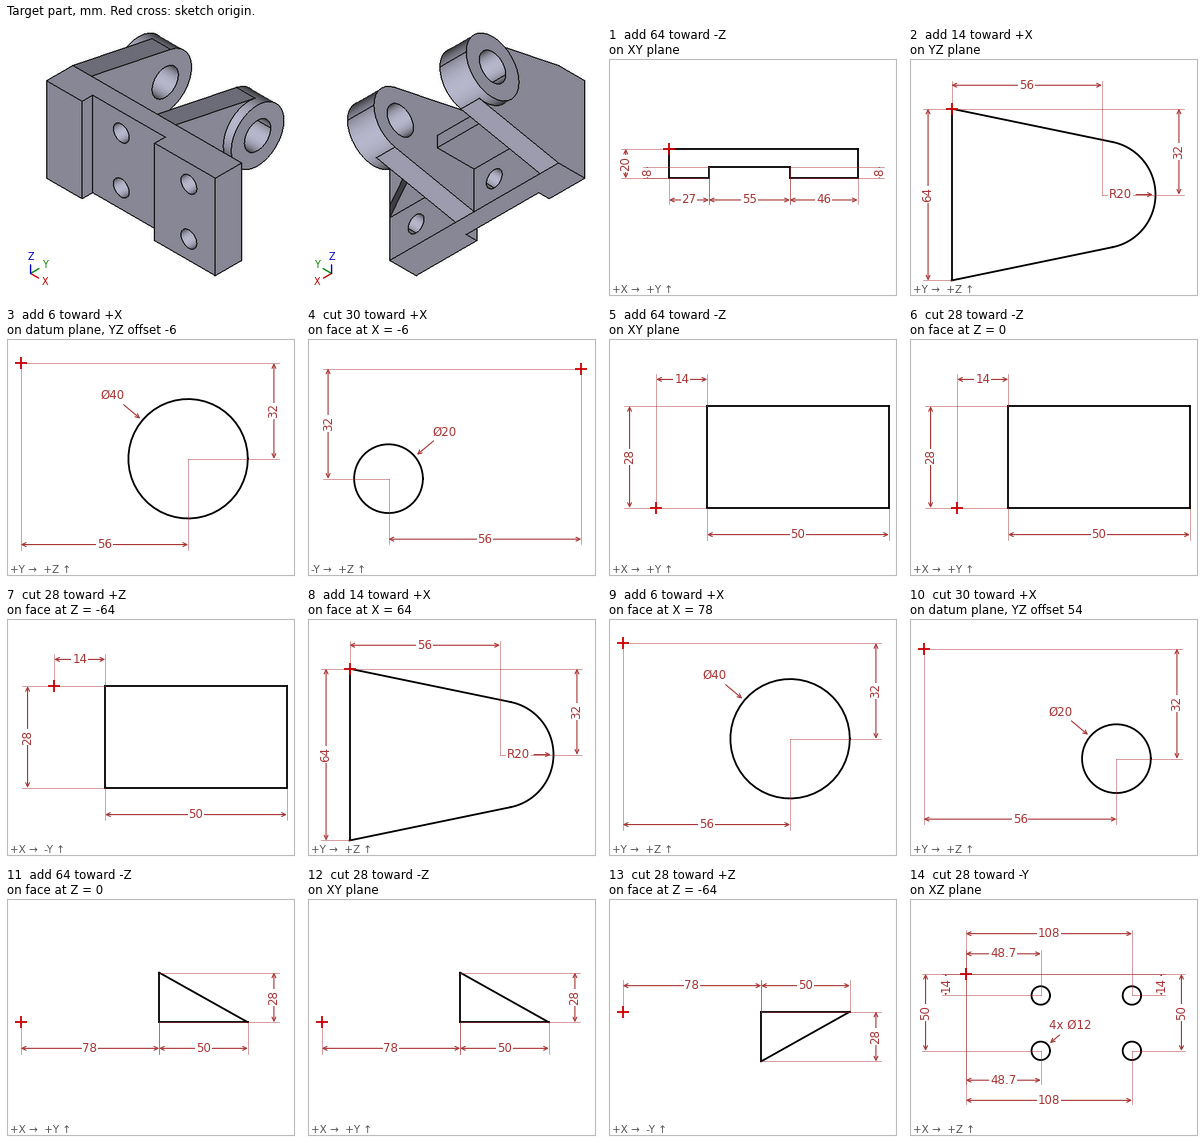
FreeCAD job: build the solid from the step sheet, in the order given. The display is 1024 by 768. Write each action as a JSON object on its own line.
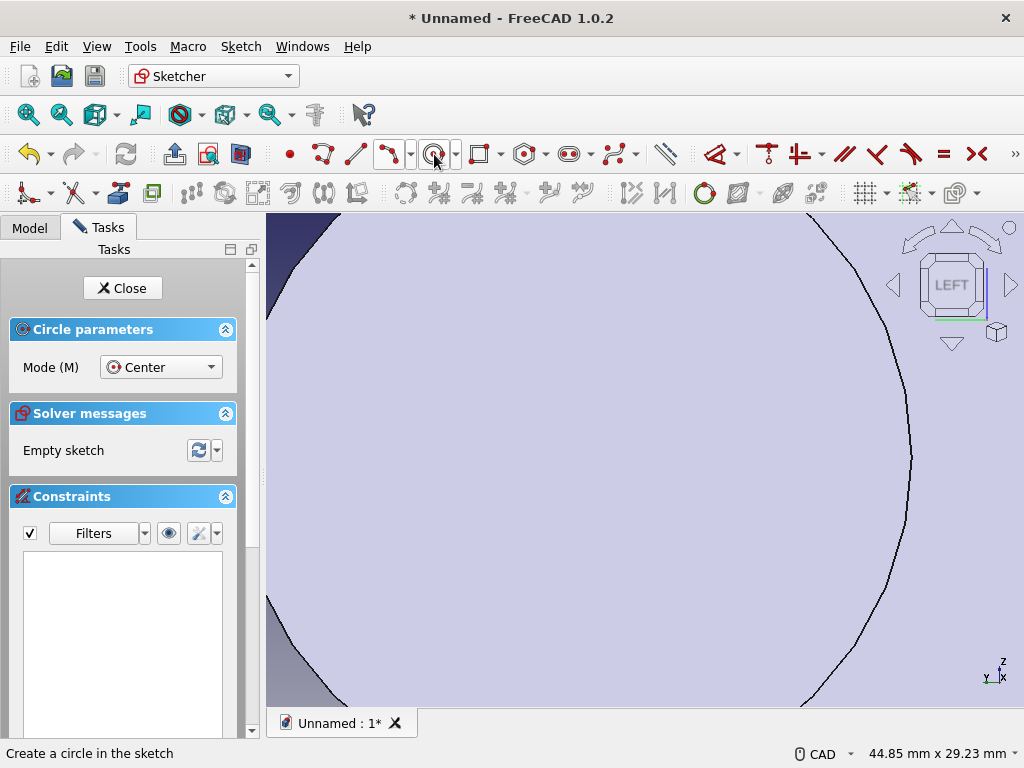
{"action": "left_click", "coordinate": [574, 457]}
{"action": "left_click", "coordinate": [693, 338]}
{"action": "key", "text": "Escape"}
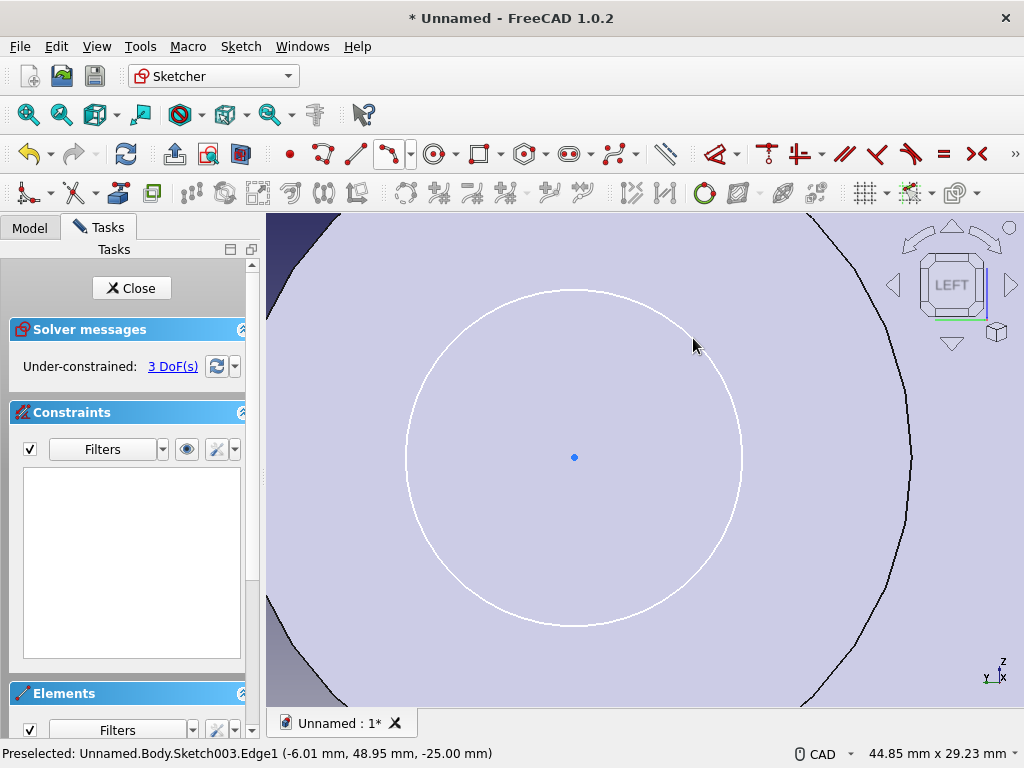
{"action": "left_click", "coordinate": [714, 154]}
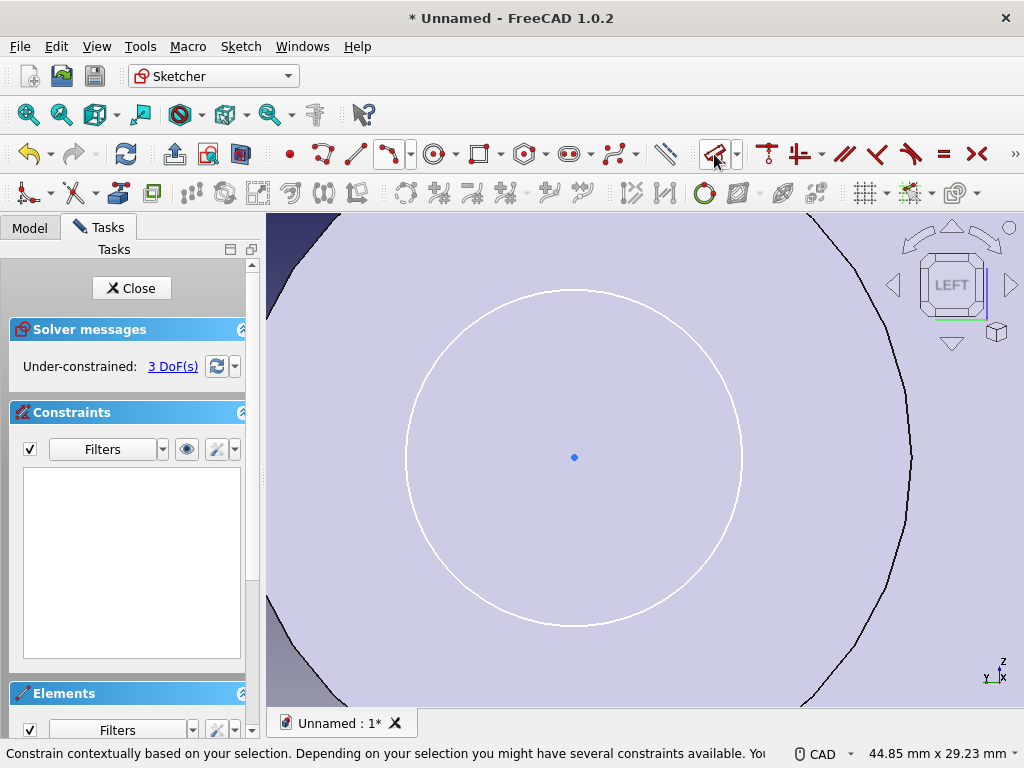
{"action": "left_click", "coordinate": [693, 339]}
{"action": "left_click", "coordinate": [716, 316]}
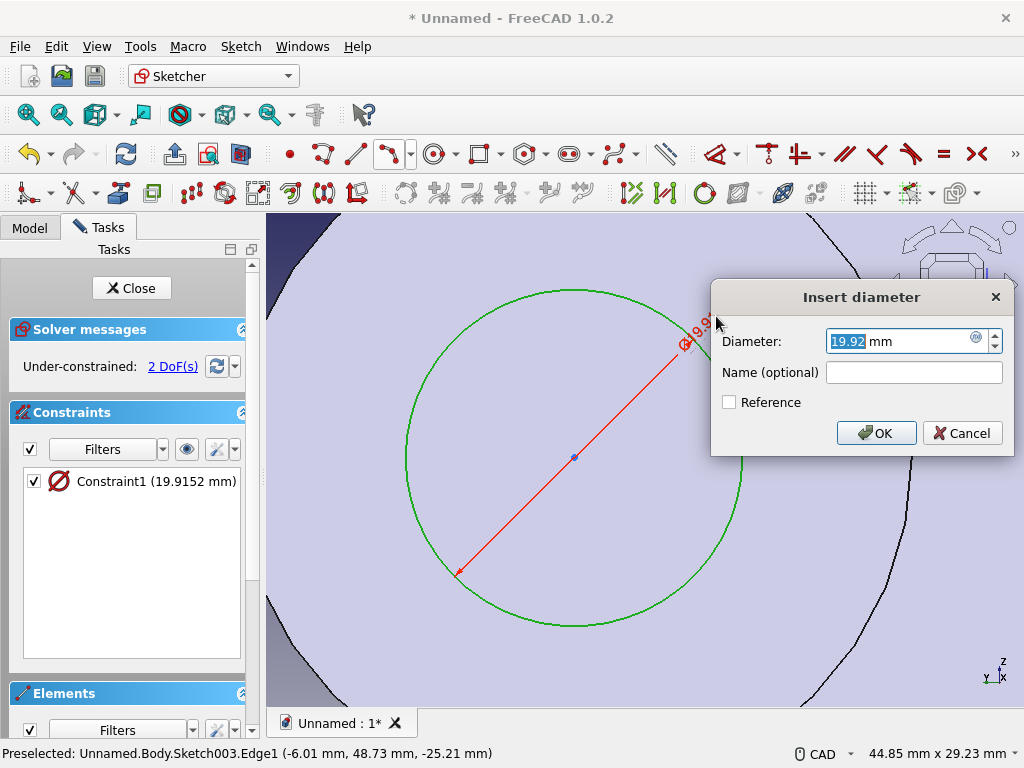
{"action": "type", "text": "20"}
{"action": "key", "text": "Return"}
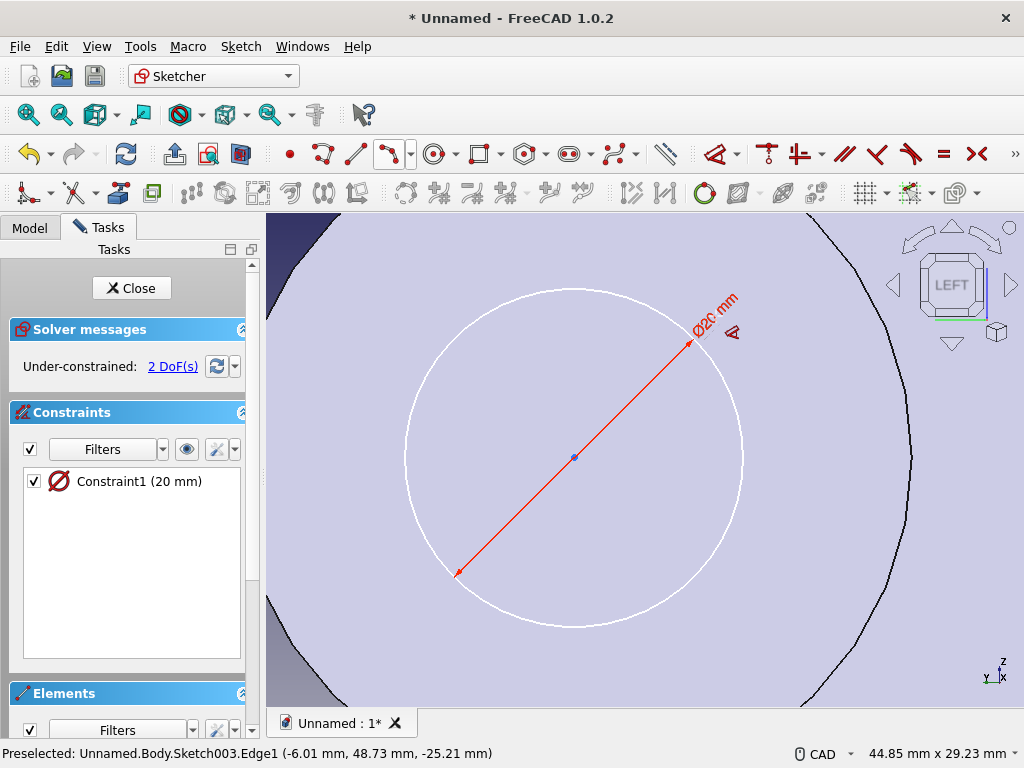
{"action": "left_click", "coordinate": [574, 458]}
{"action": "left_click", "coordinate": [716, 492]}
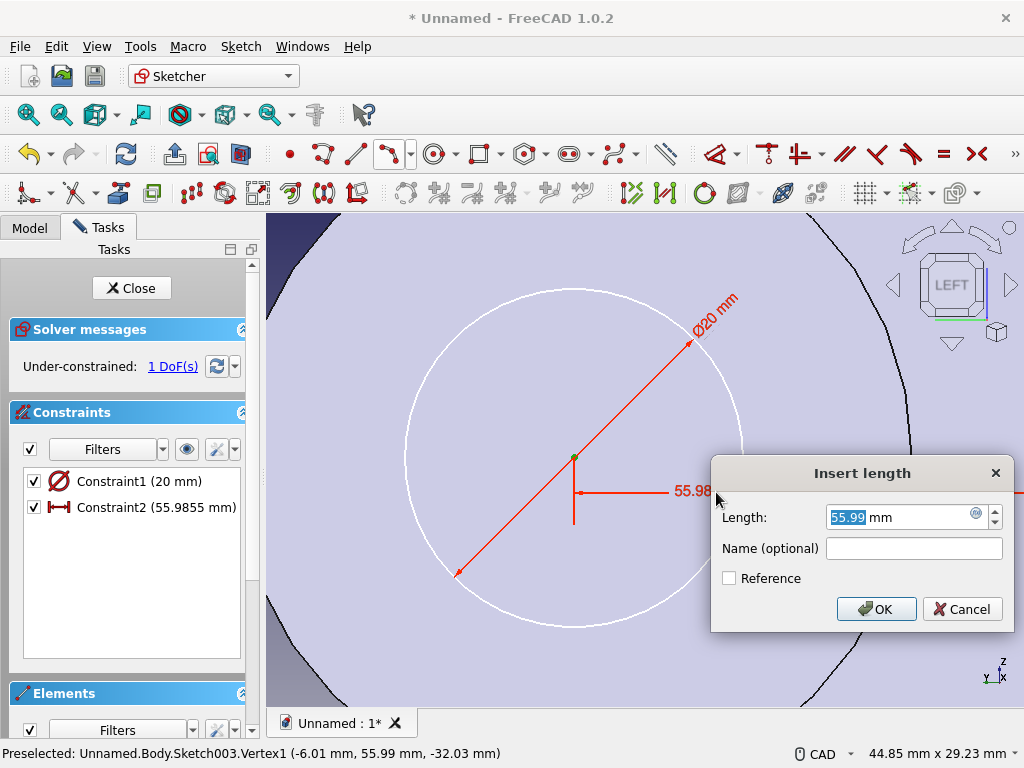
{"action": "type", "text": "56"}
{"action": "key", "text": "Return"}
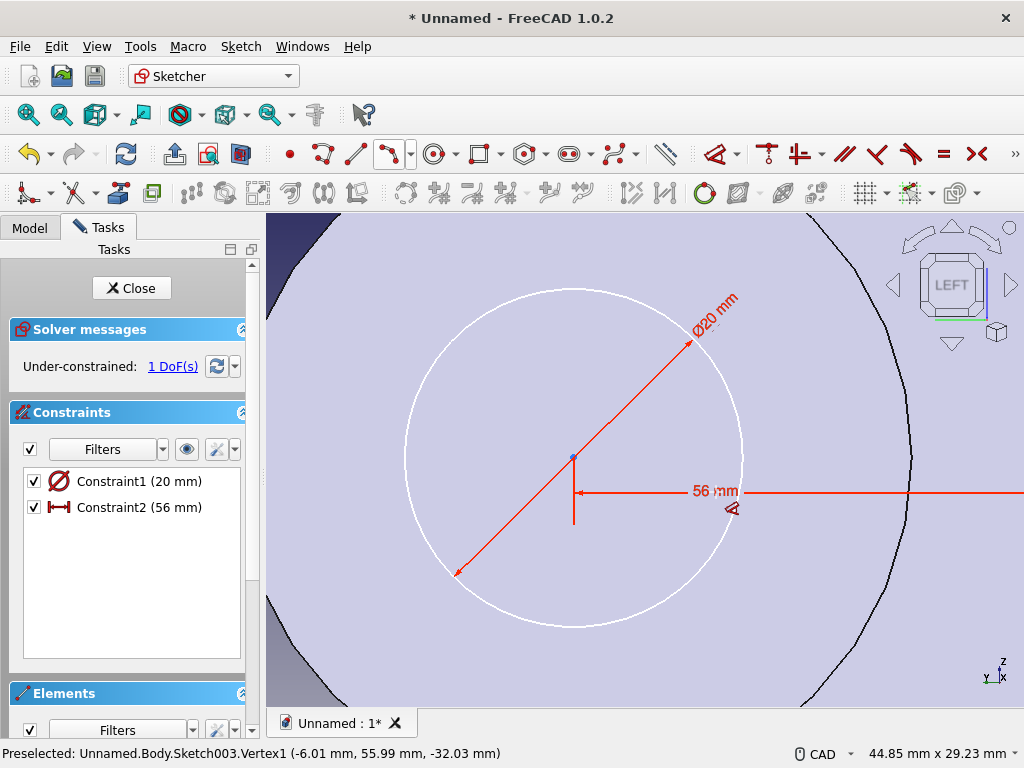
{"action": "left_click", "coordinate": [574, 458]}
{"action": "left_click", "coordinate": [540, 349]}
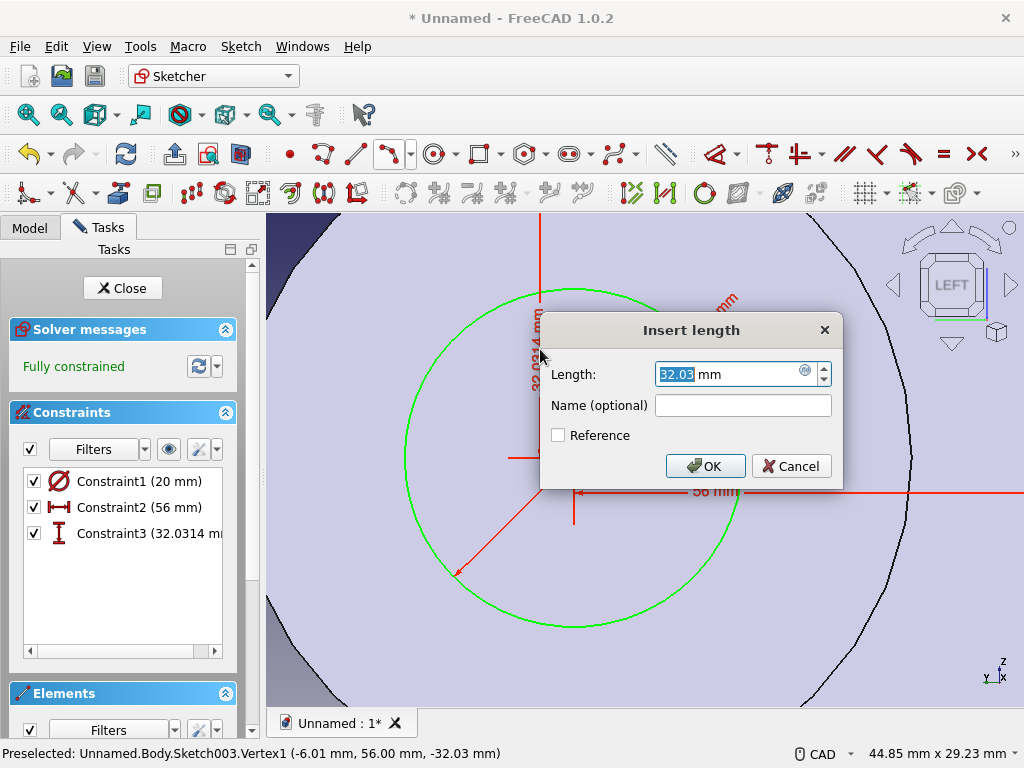
{"action": "type", "text": "32"}
{"action": "key", "text": "Return"}
{"action": "key", "text": "Escape"}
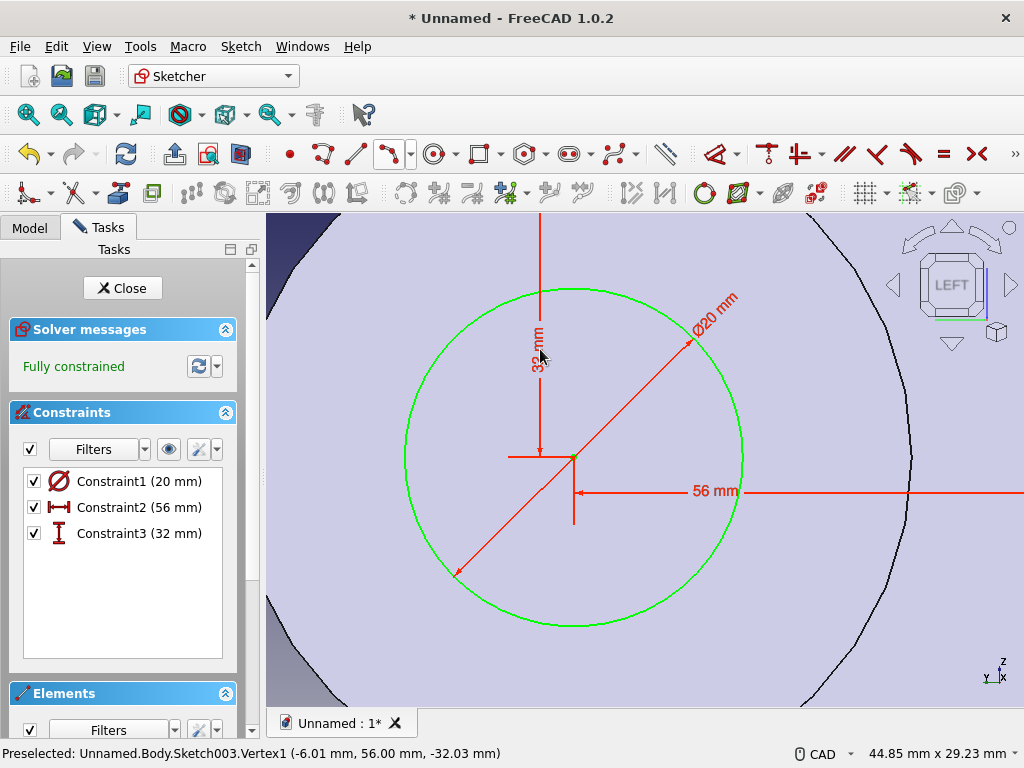
{"action": "left_click", "coordinate": [123, 288]}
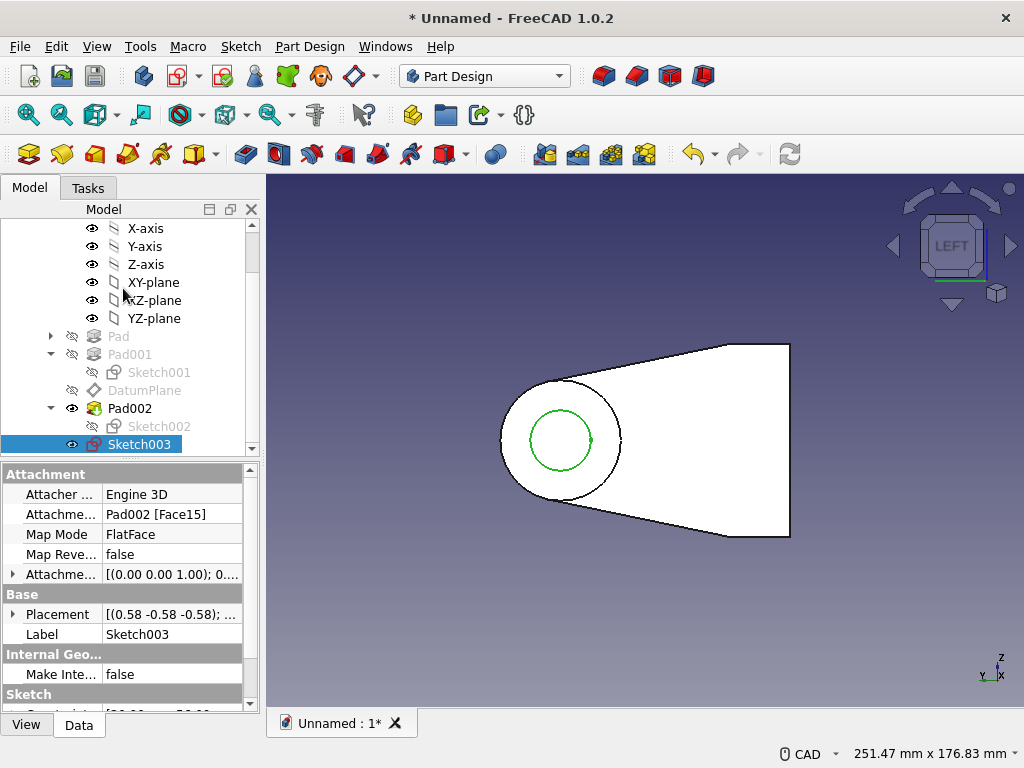
{"action": "left_click", "coordinate": [246, 154]}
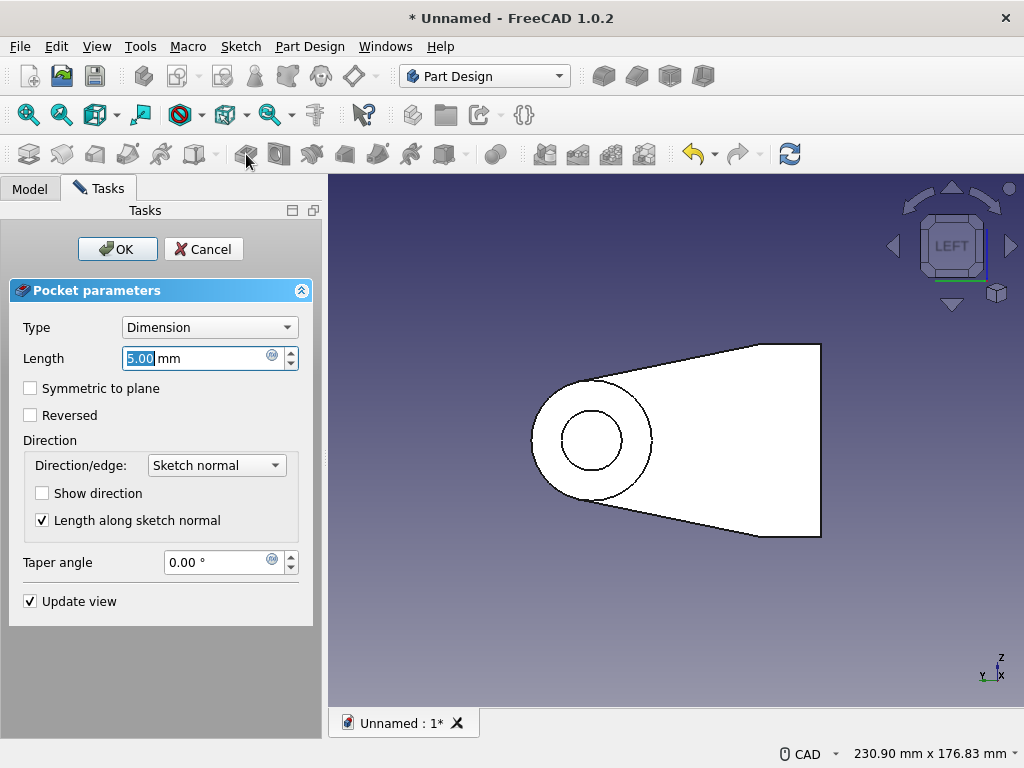
{"action": "type", "text": "30"}
{"action": "key", "text": "Tab"}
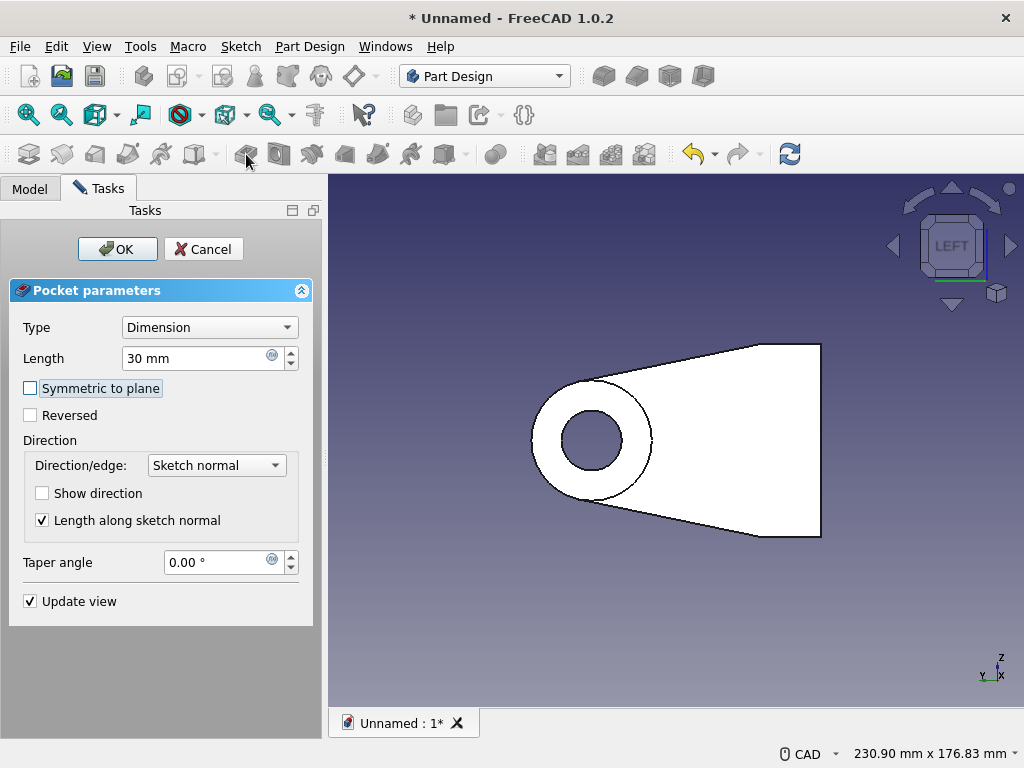
{"action": "left_click", "coordinate": [118, 249]}